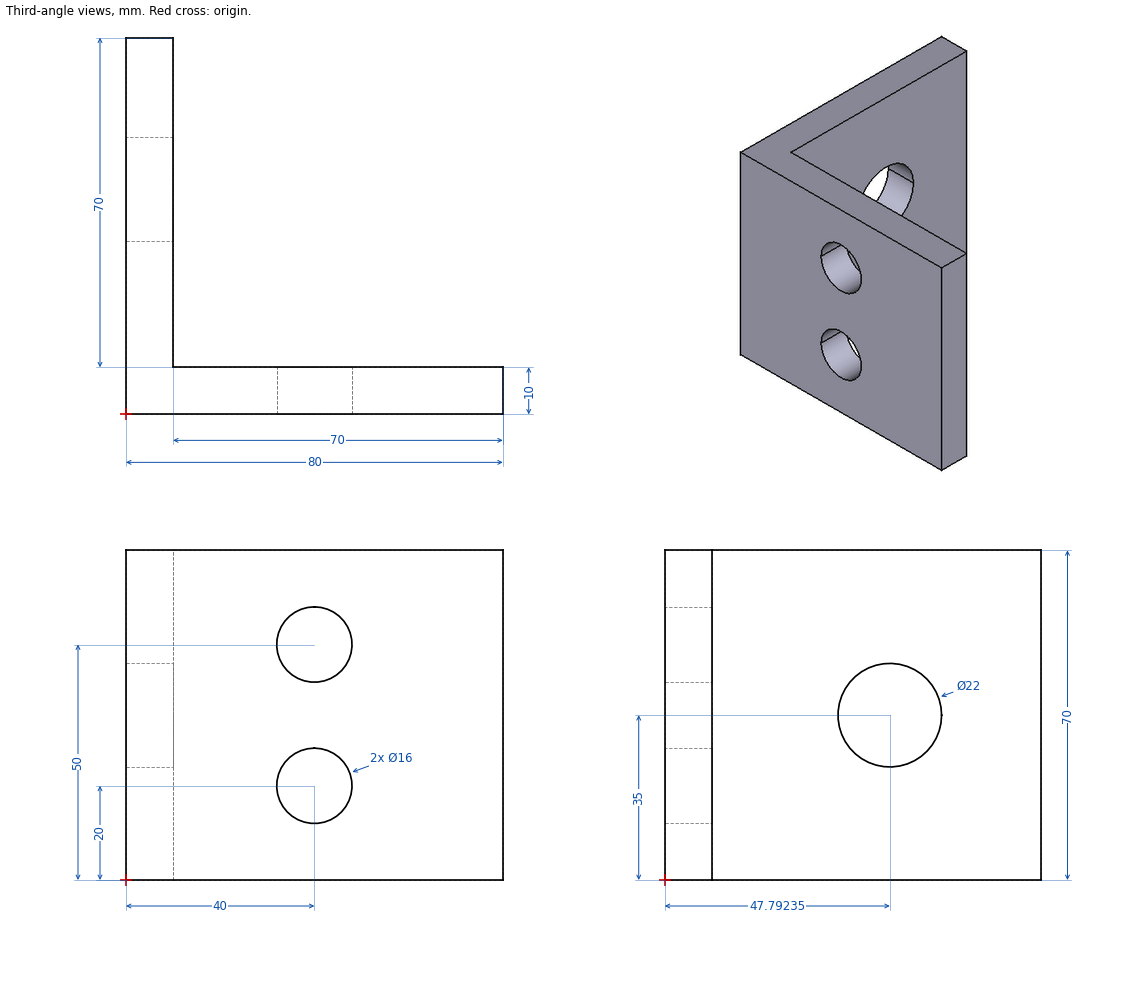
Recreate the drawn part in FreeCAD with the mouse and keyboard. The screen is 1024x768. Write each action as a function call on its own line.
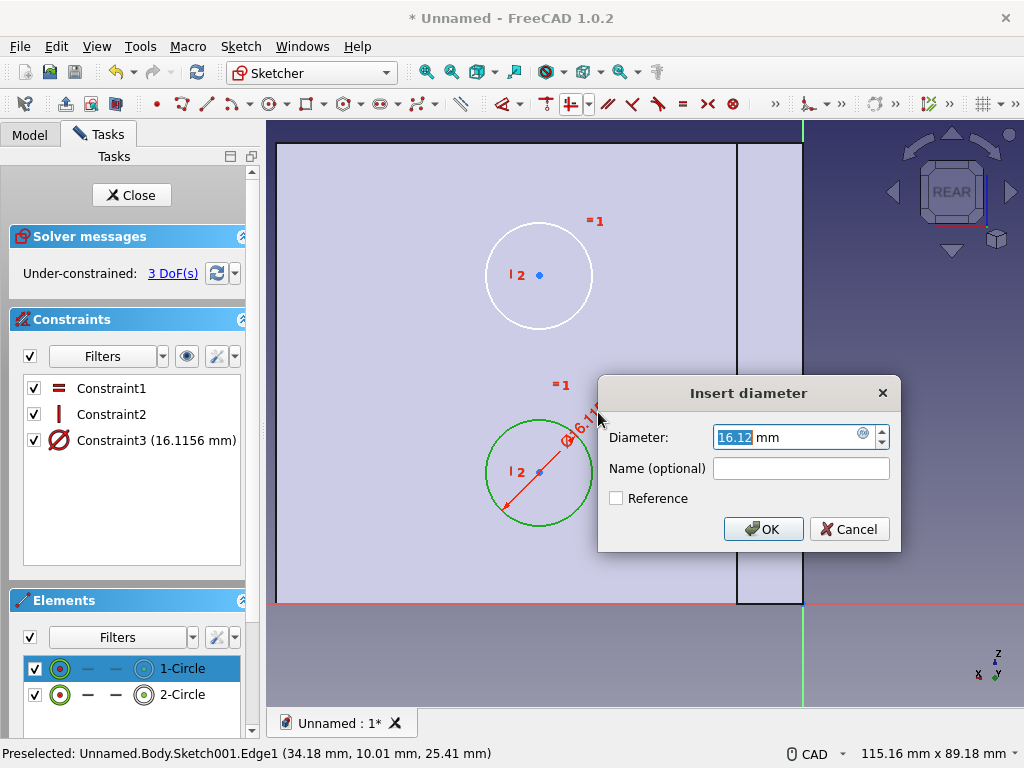
text(16)
key(Return)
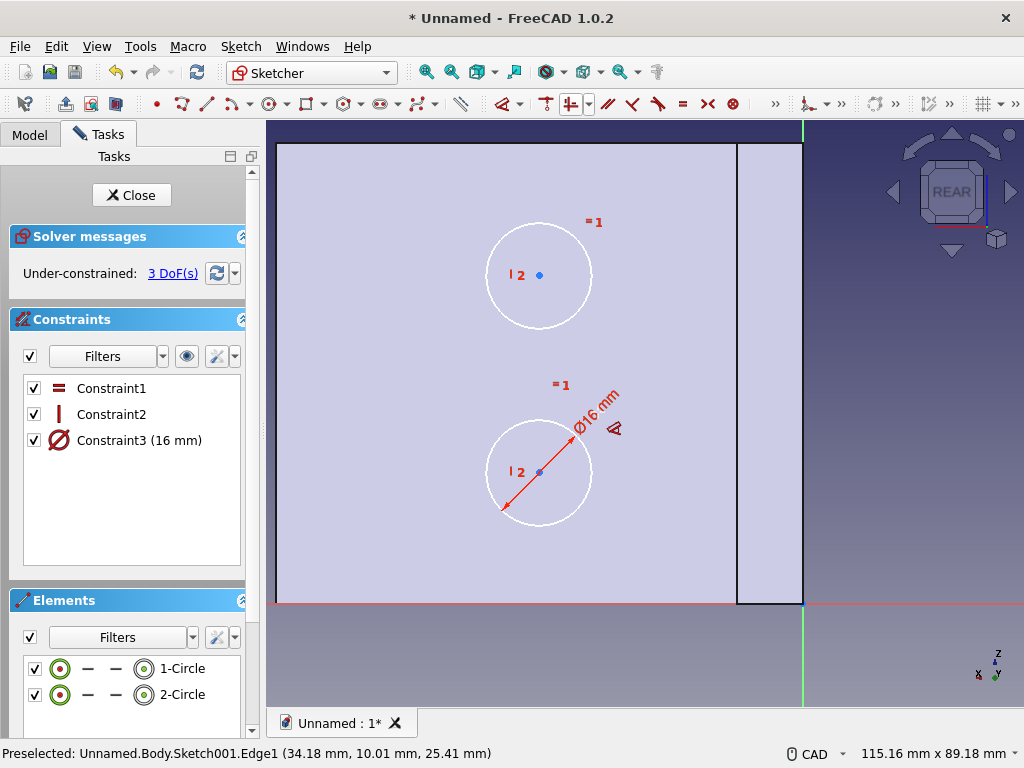
click(539, 473)
click(671, 638)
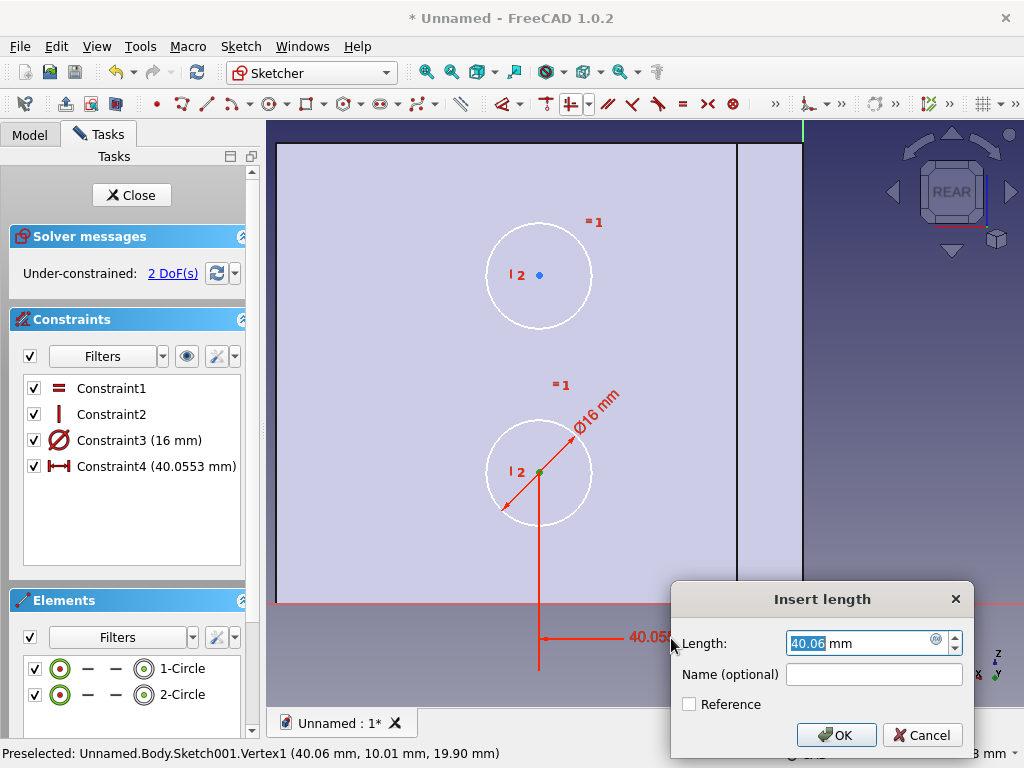
text(40)
key(Return)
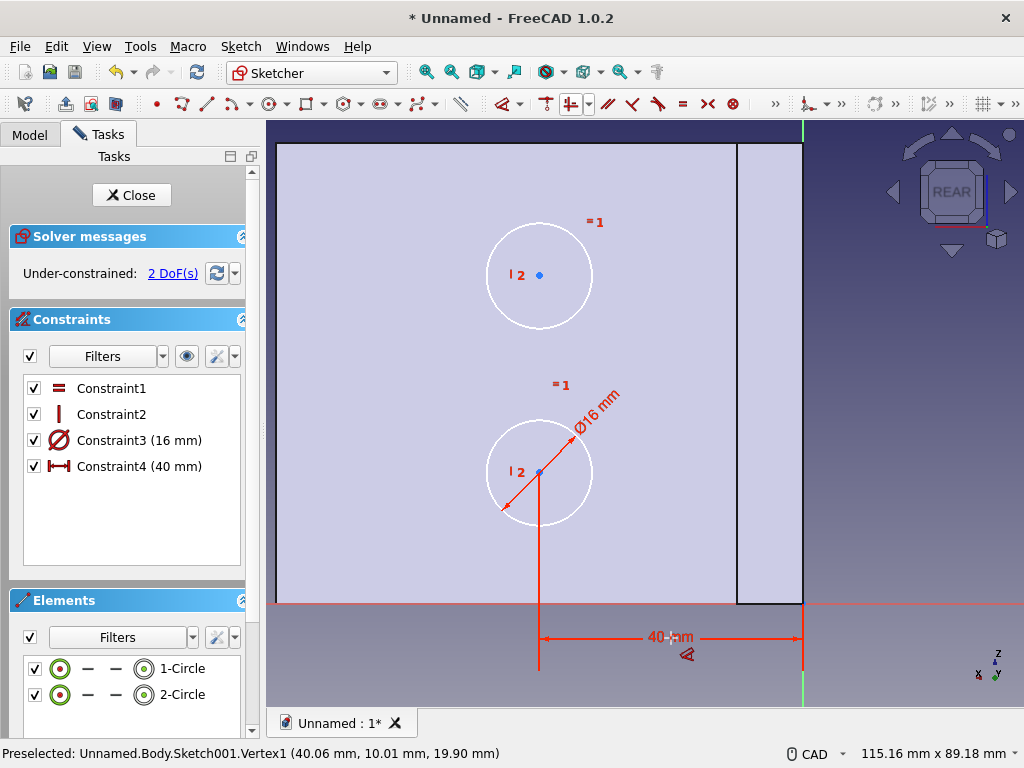
click(539, 473)
click(837, 538)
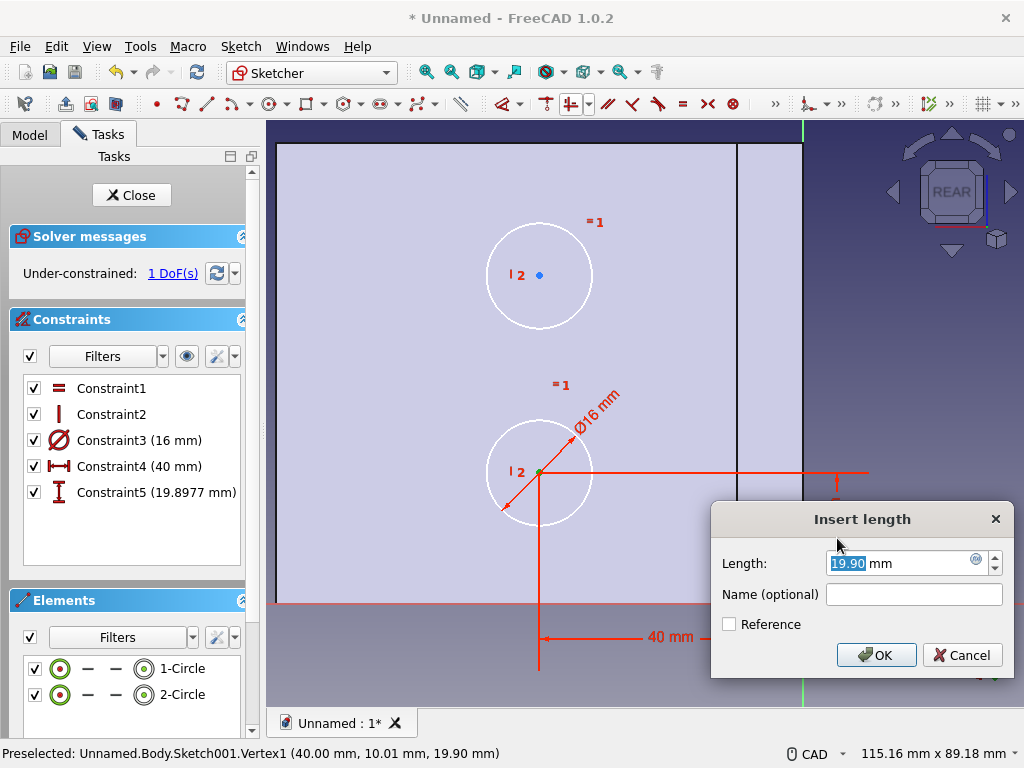
text(20)
key(Return)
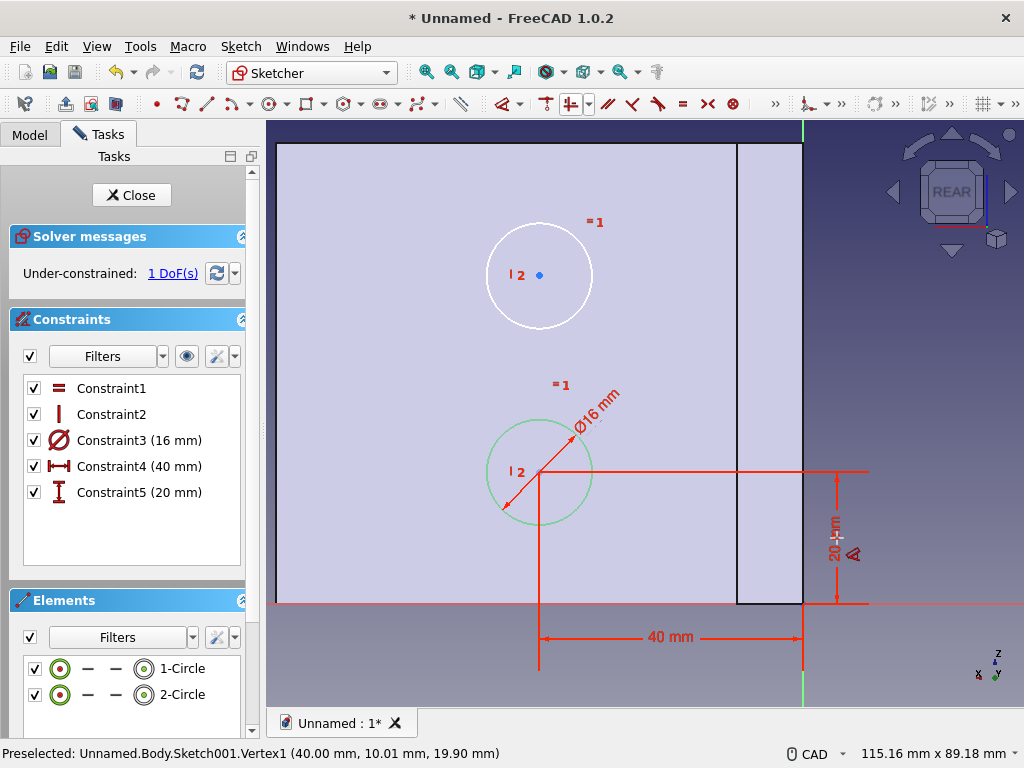
click(539, 276)
click(837, 440)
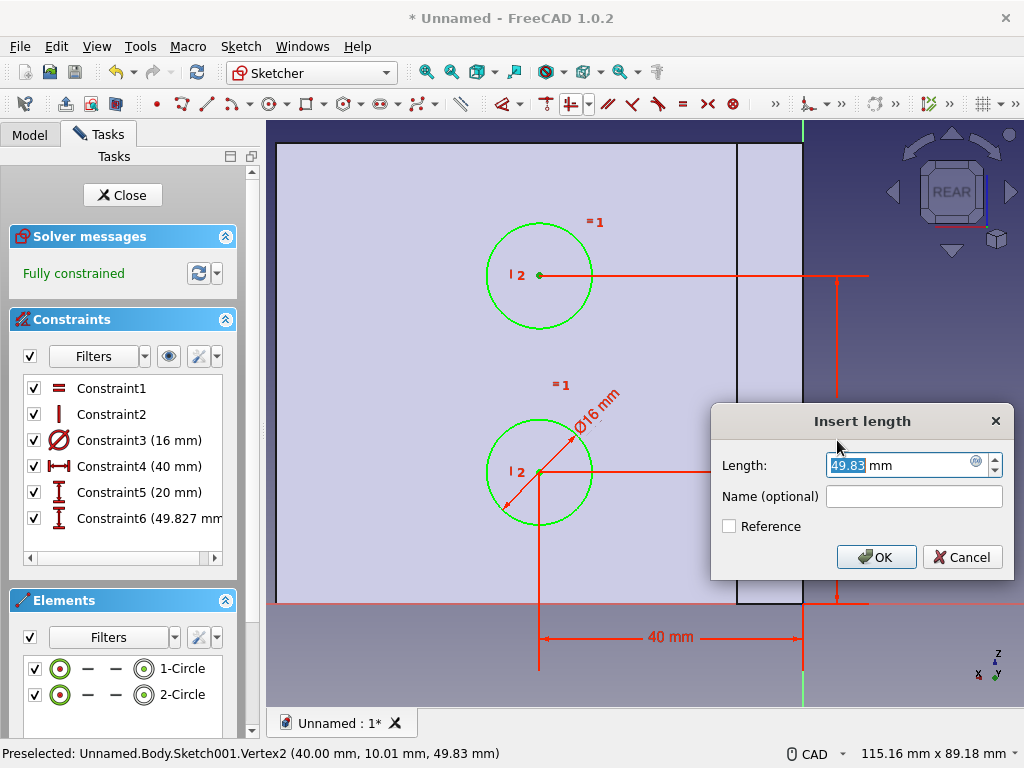
text(50)
key(Return)
key(Escape)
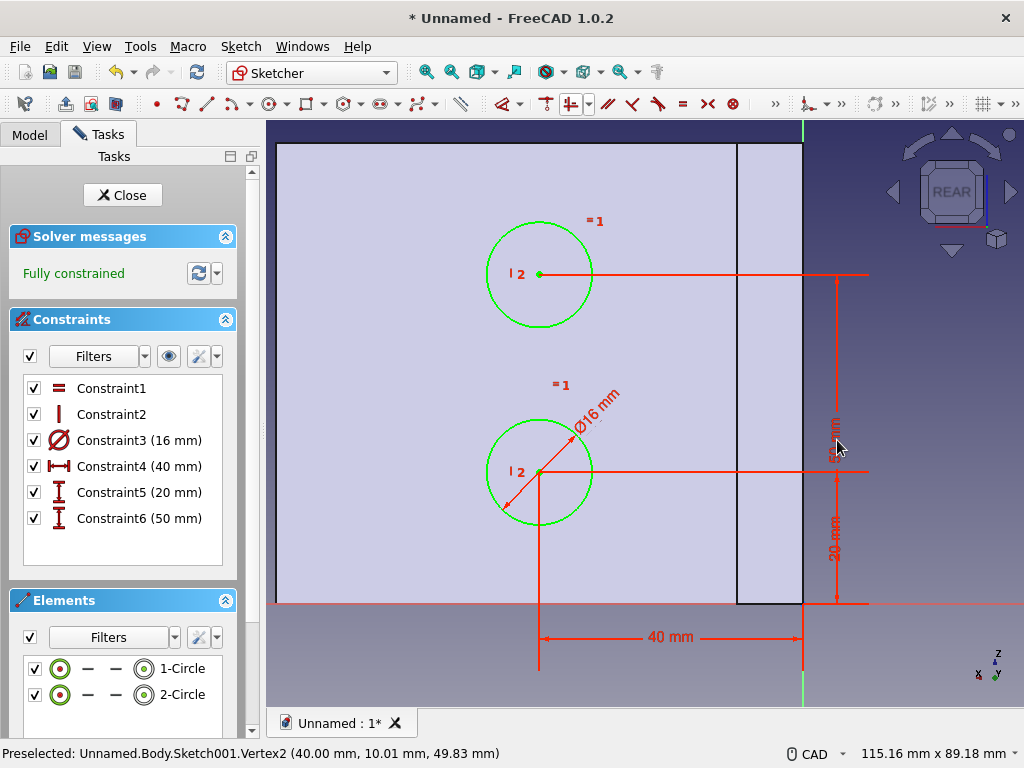
click(123, 195)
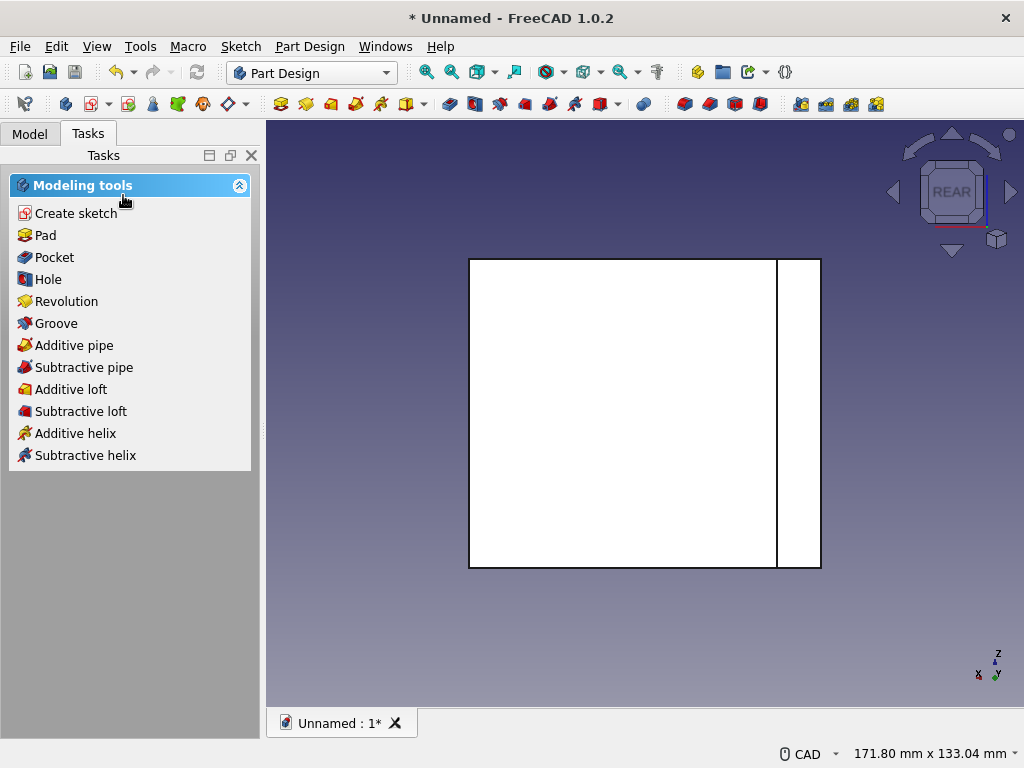
click(450, 104)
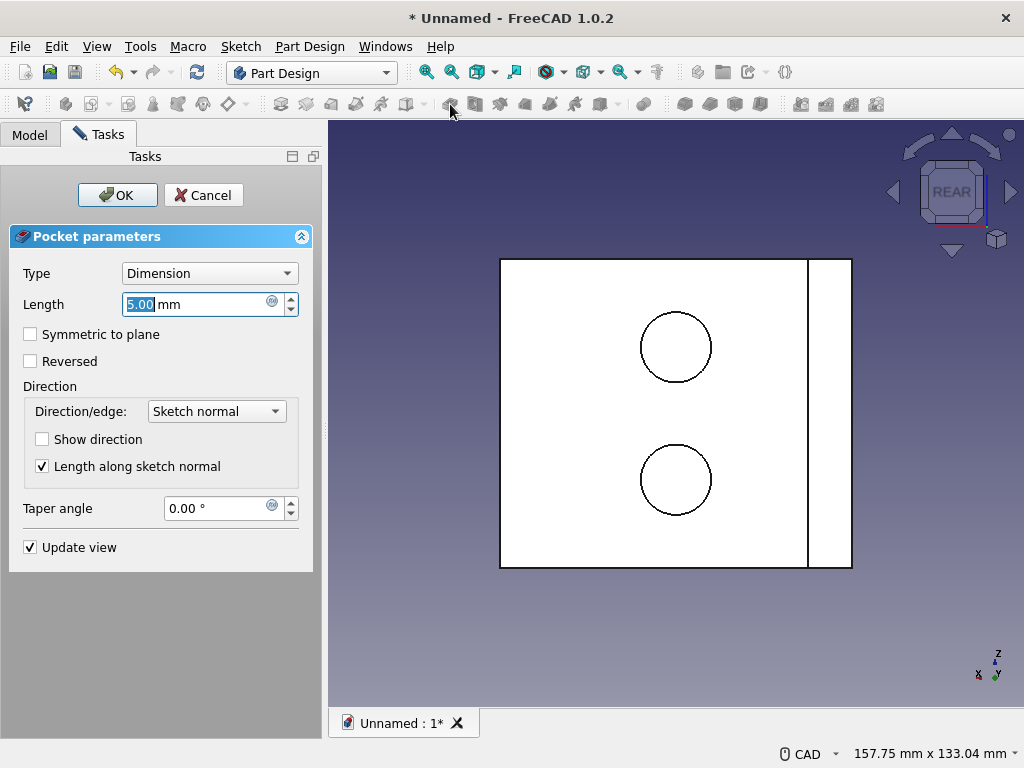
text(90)
key(Tab)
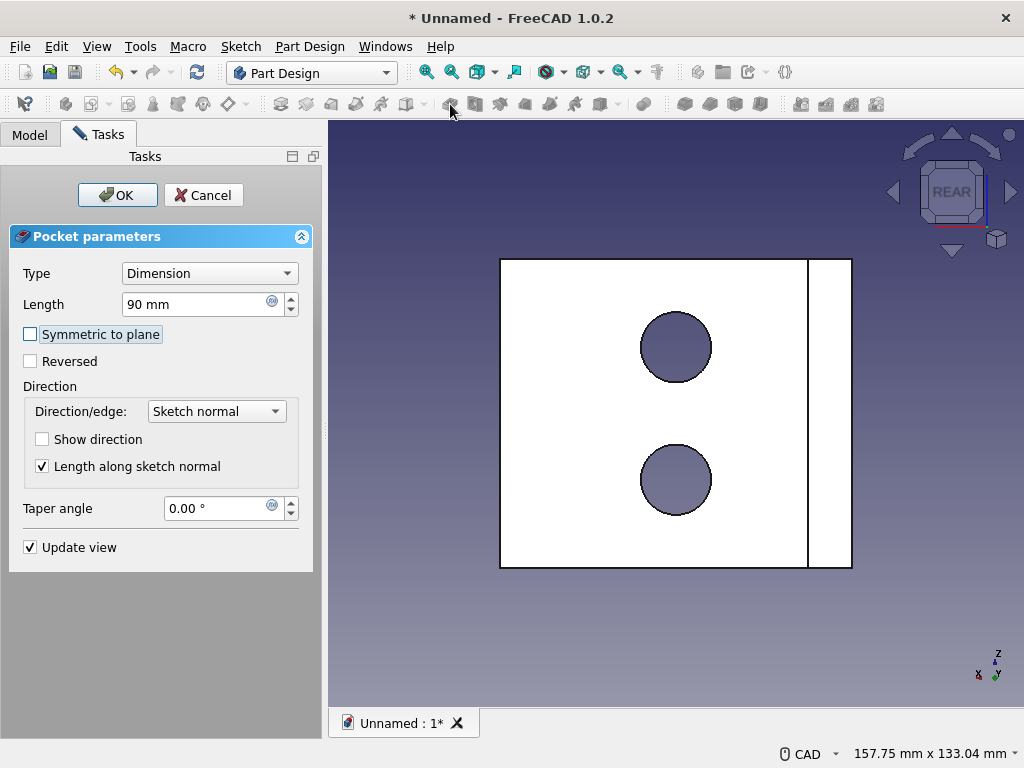
click(118, 195)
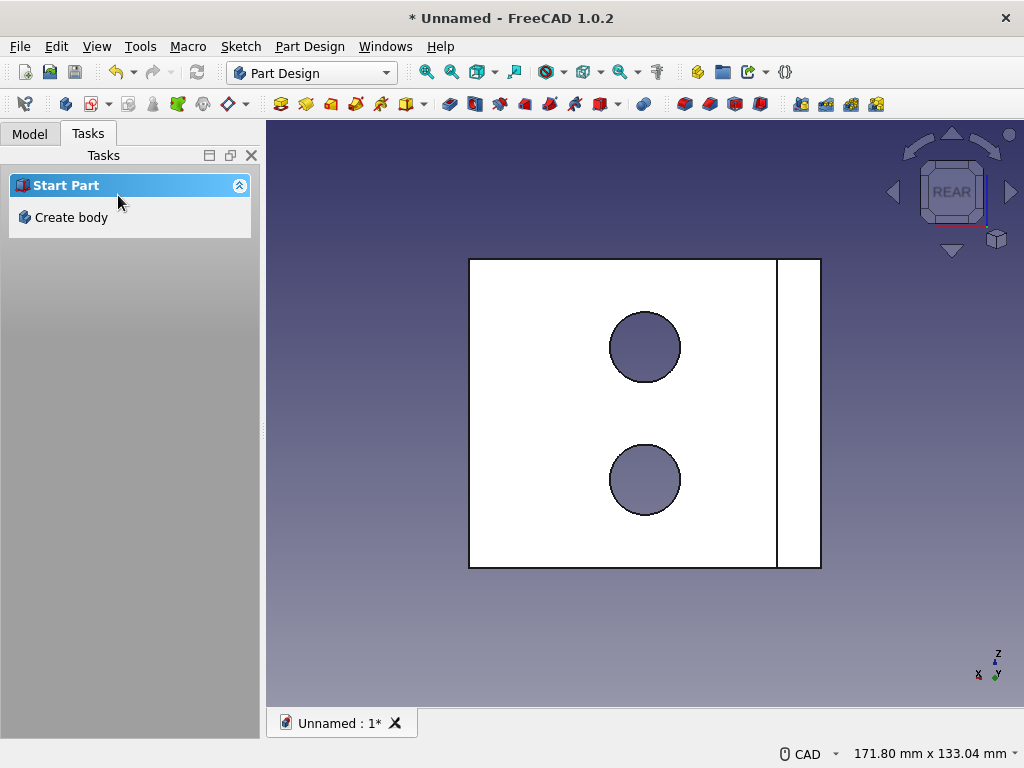
key(0)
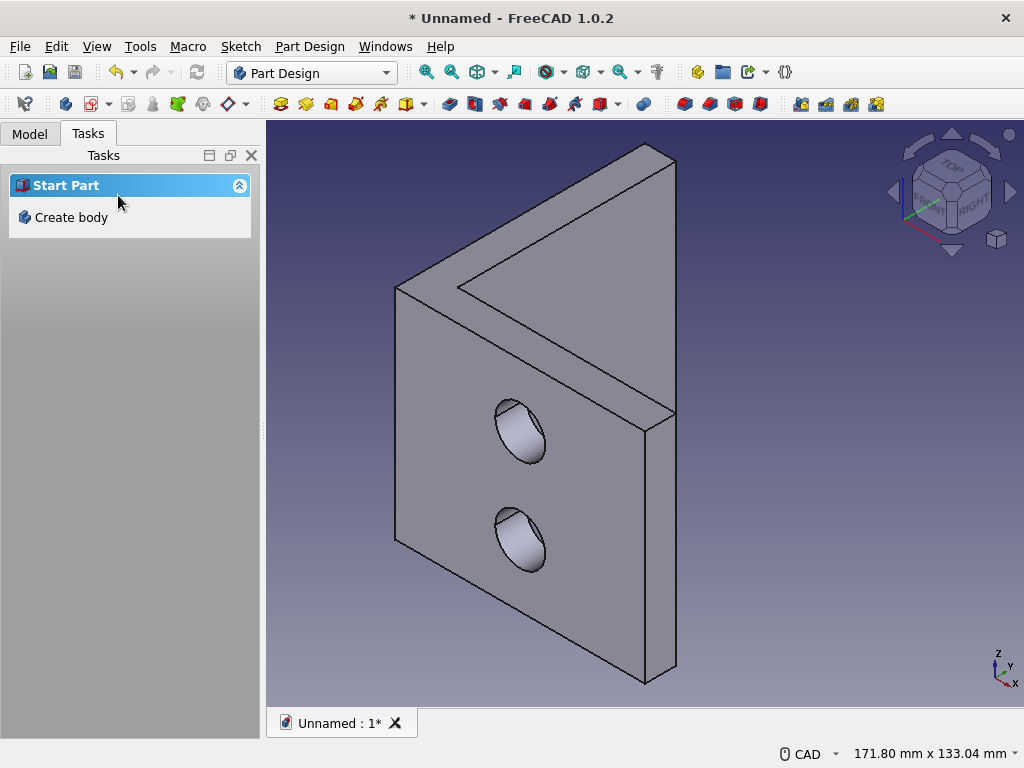
click(598, 295)